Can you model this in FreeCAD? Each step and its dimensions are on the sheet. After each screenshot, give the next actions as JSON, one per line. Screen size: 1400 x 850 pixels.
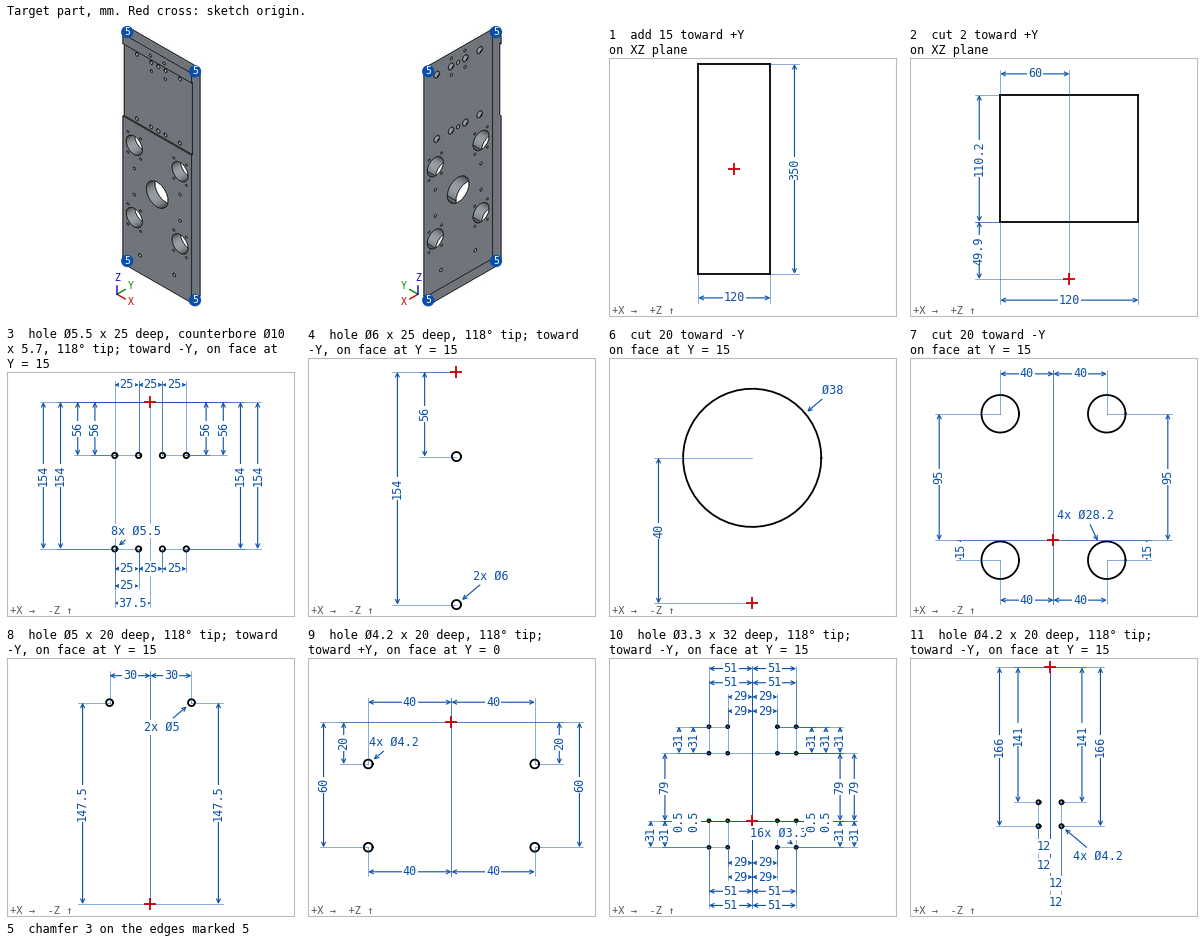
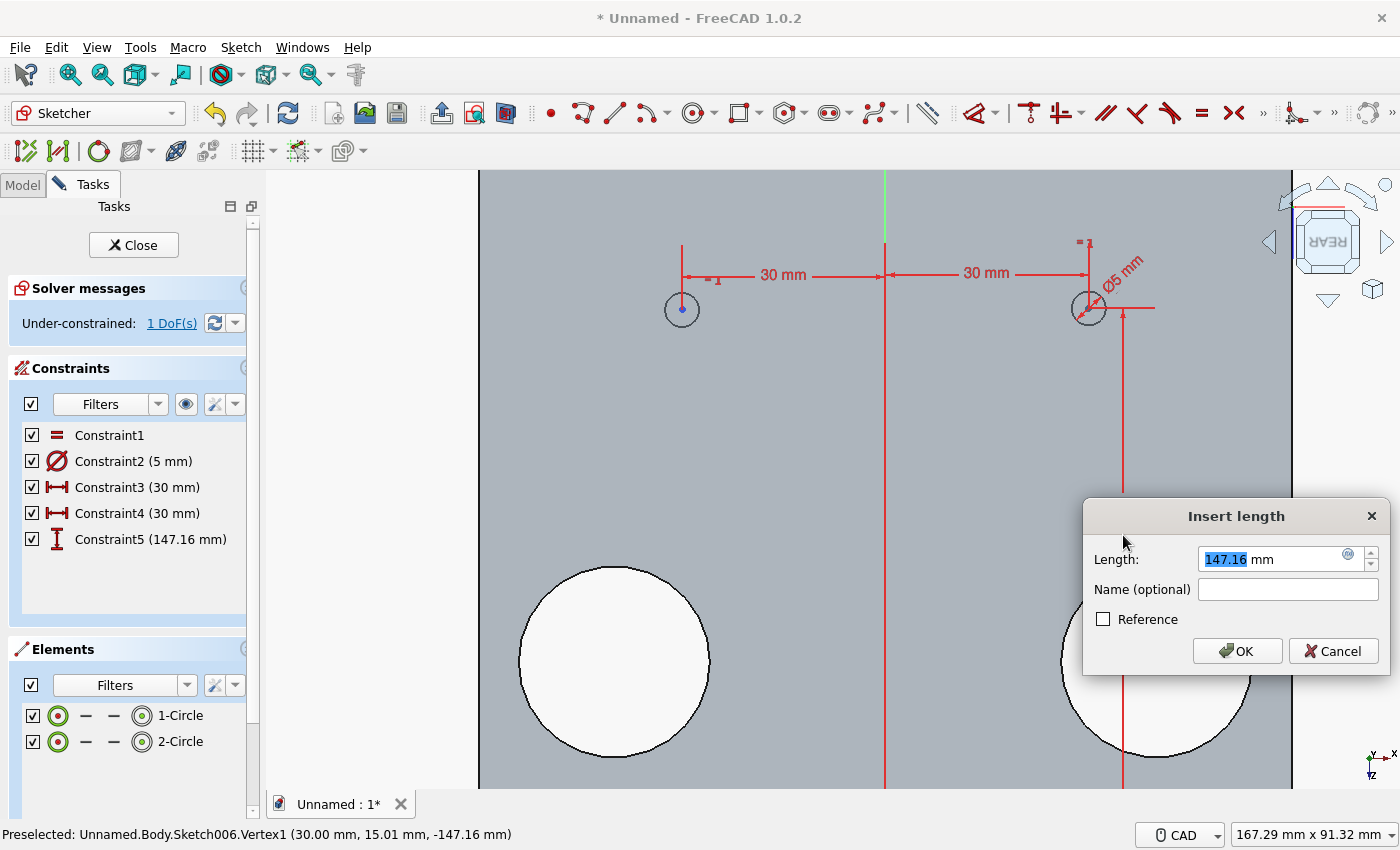
{"action": "type", "text": "147.5"}
{"action": "key", "text": "Return"}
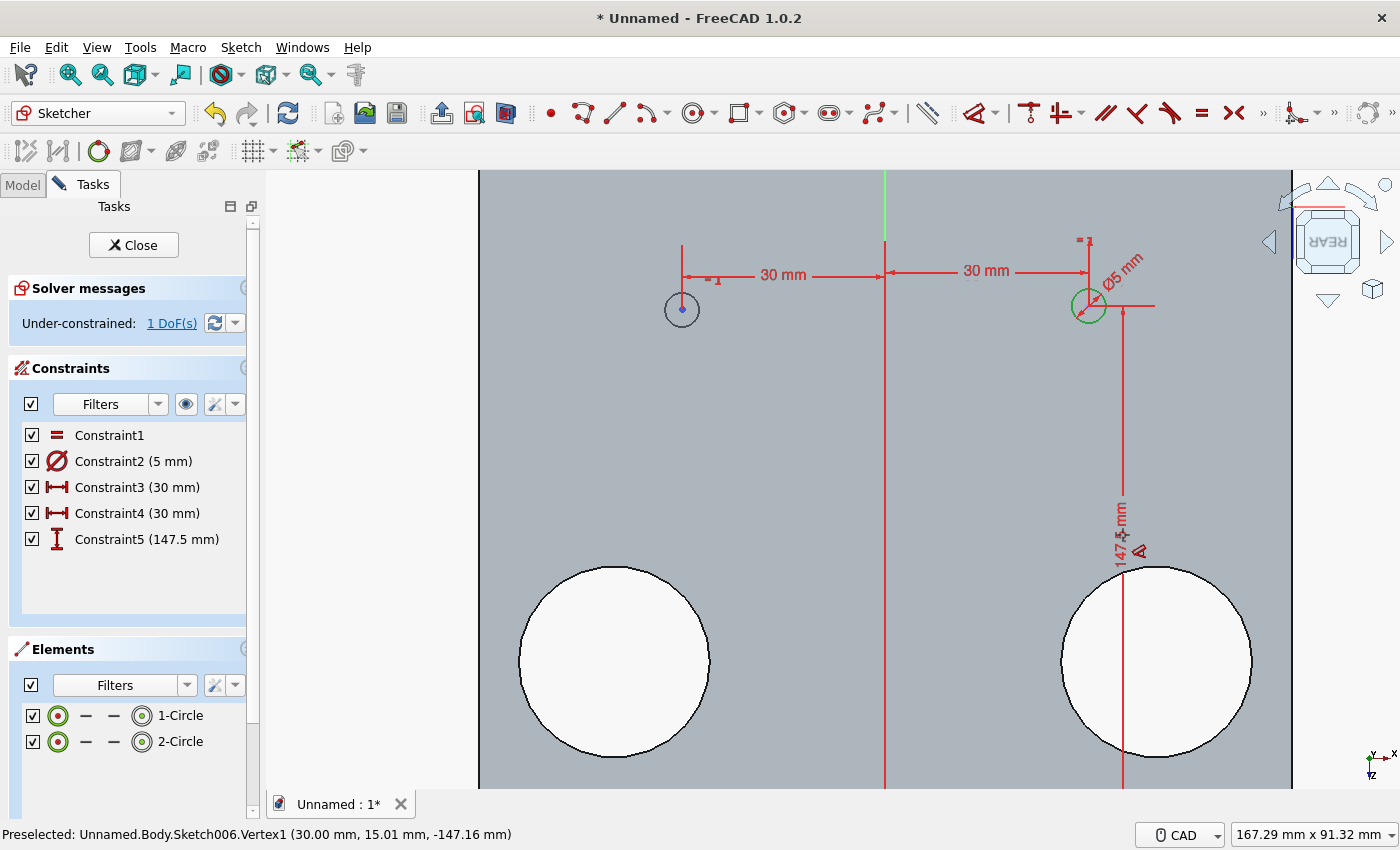
{"action": "left_click", "coordinate": [682, 310]}
{"action": "left_click", "coordinate": [648, 535]}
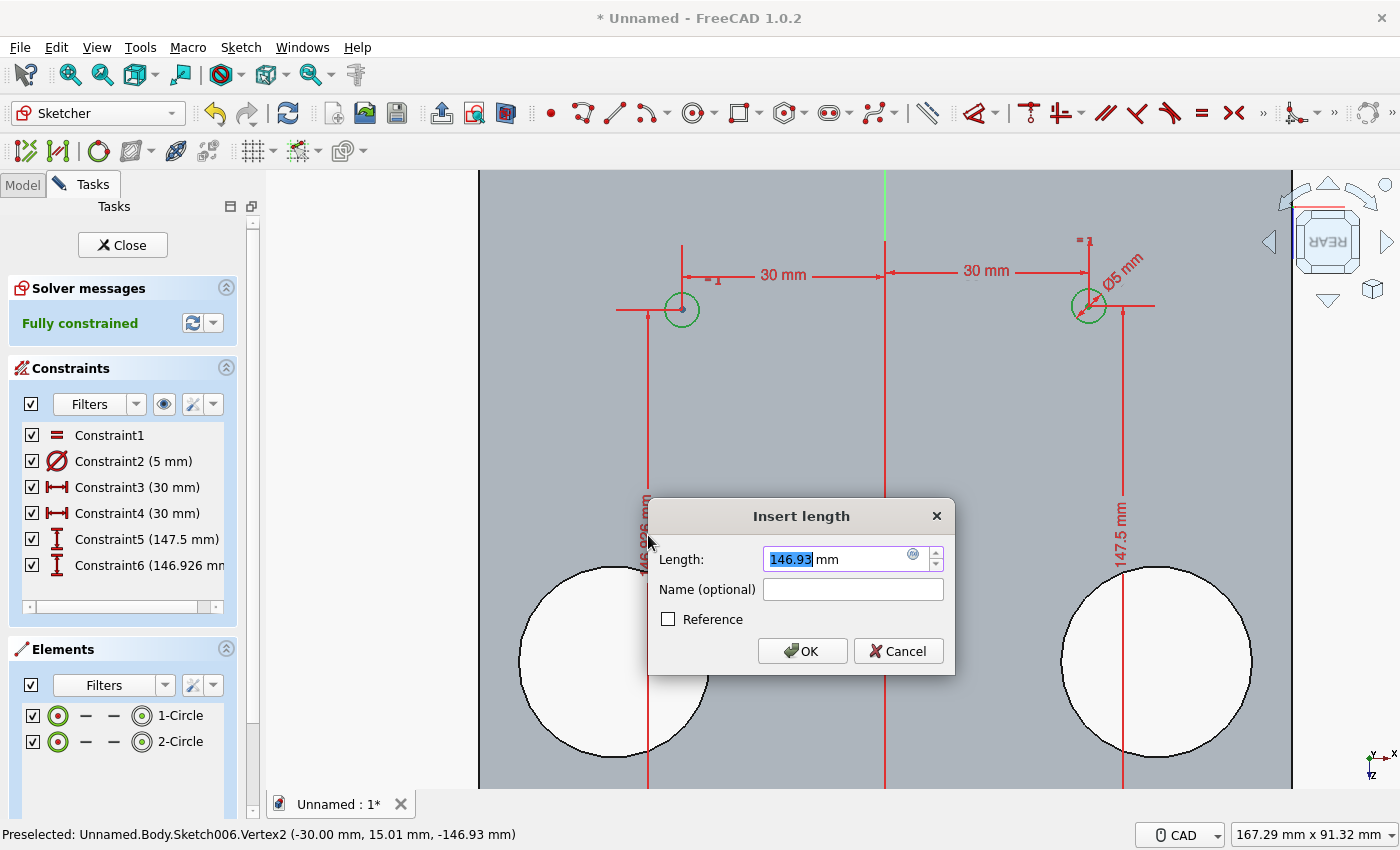
{"action": "type", "text": "147.5"}
{"action": "key", "text": "Return"}
{"action": "key", "text": "Escape"}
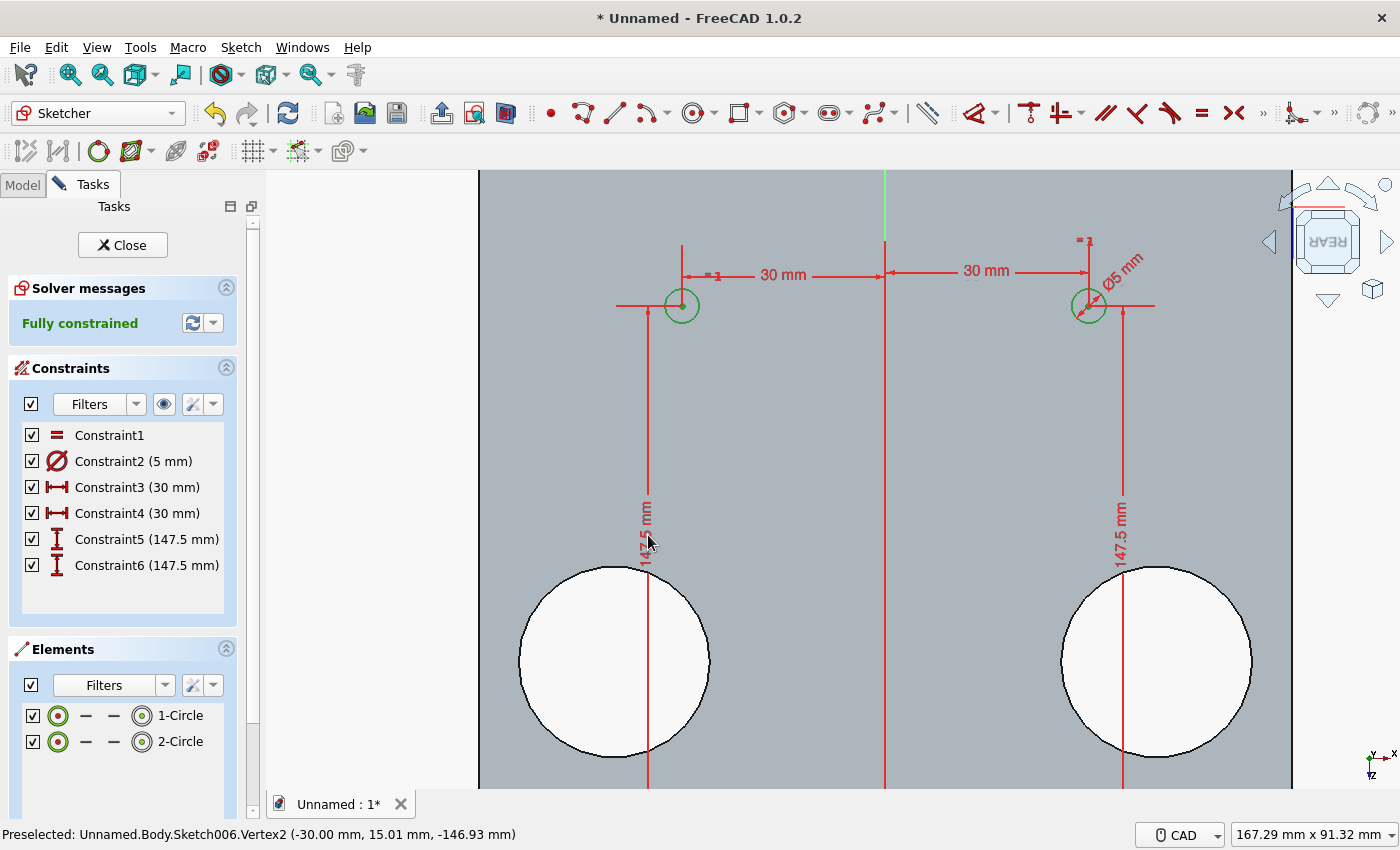
{"action": "left_click", "coordinate": [123, 245]}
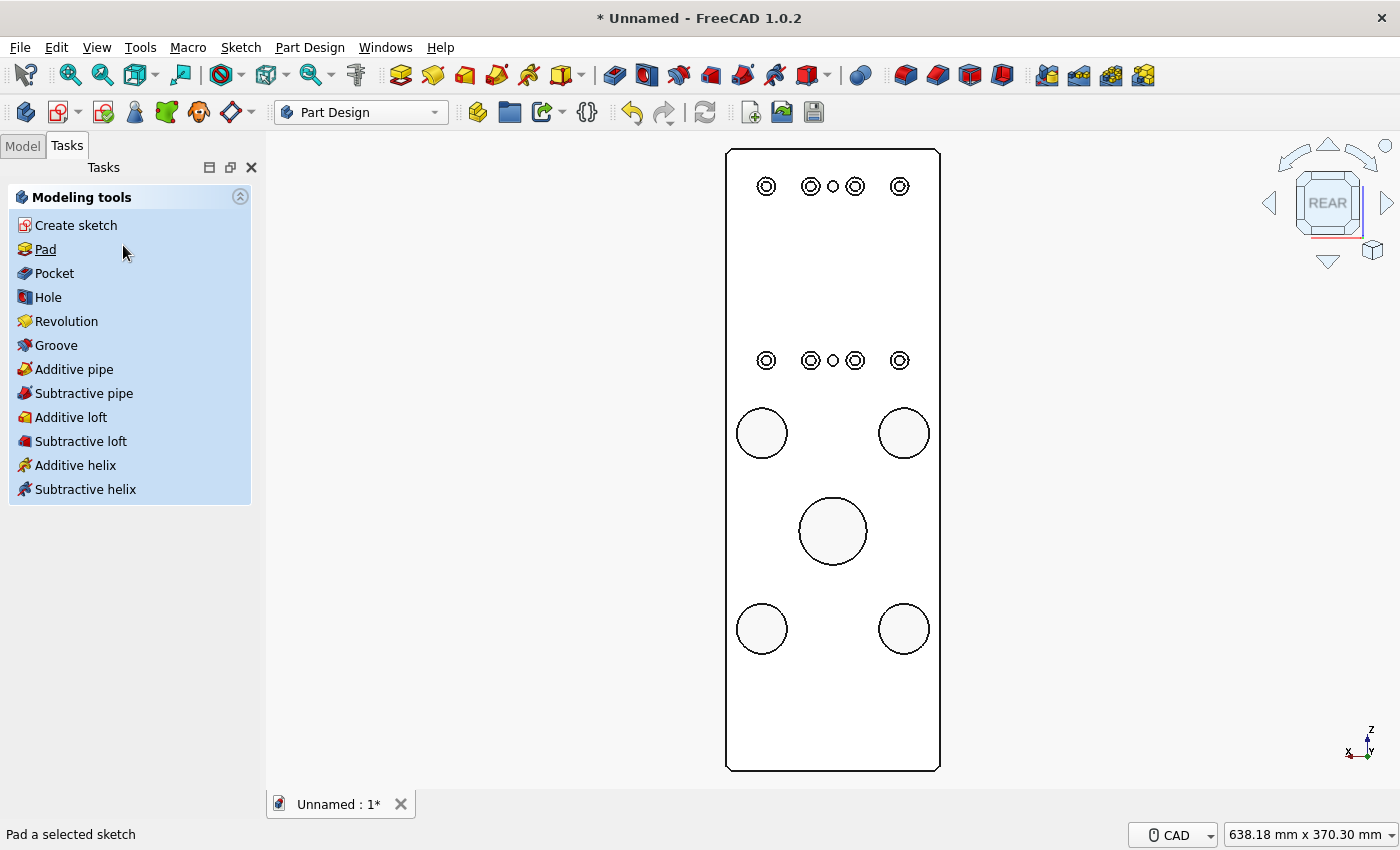
{"action": "left_click", "coordinate": [648, 76]}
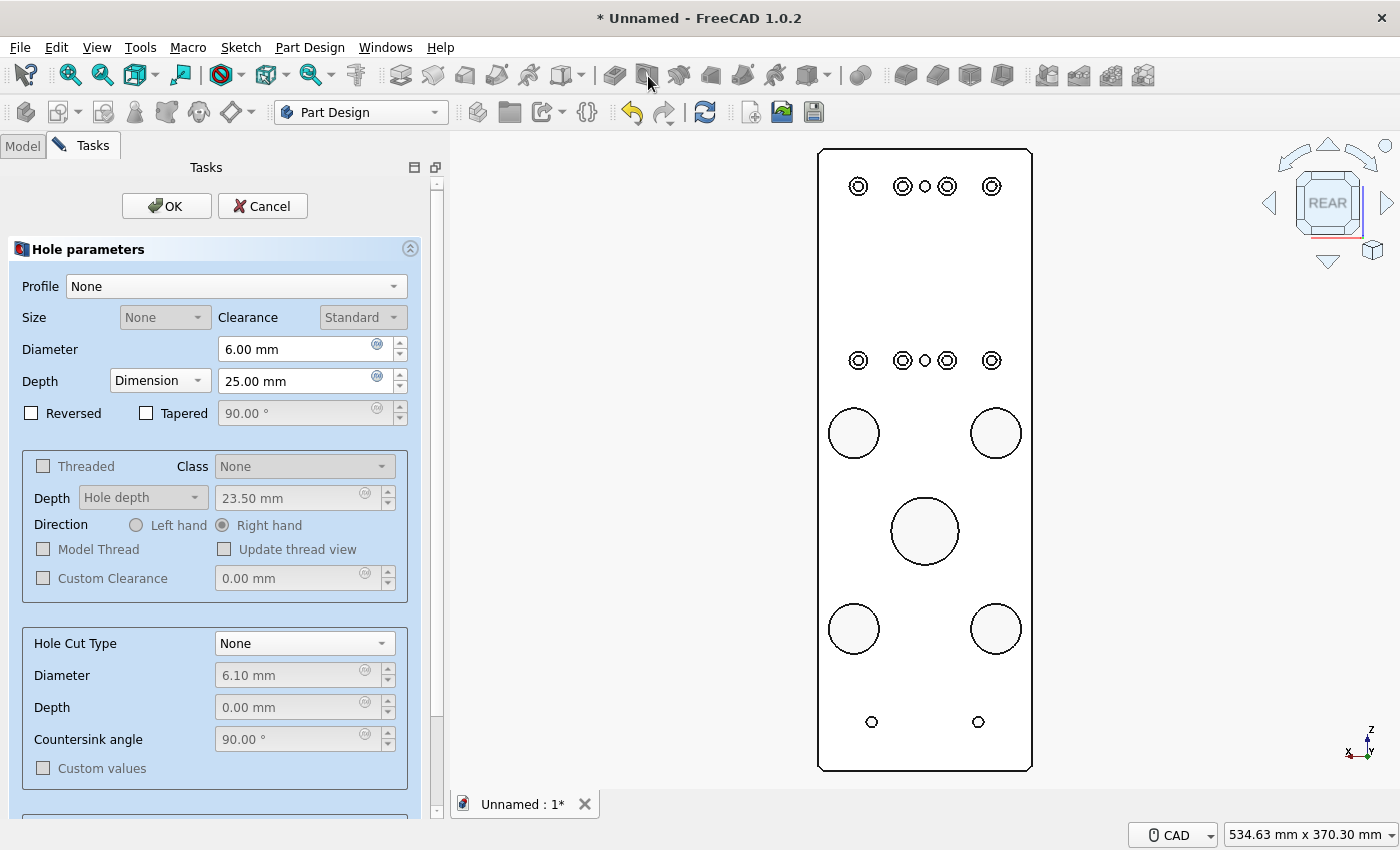
{"action": "triple_click", "coordinate": [305, 349]}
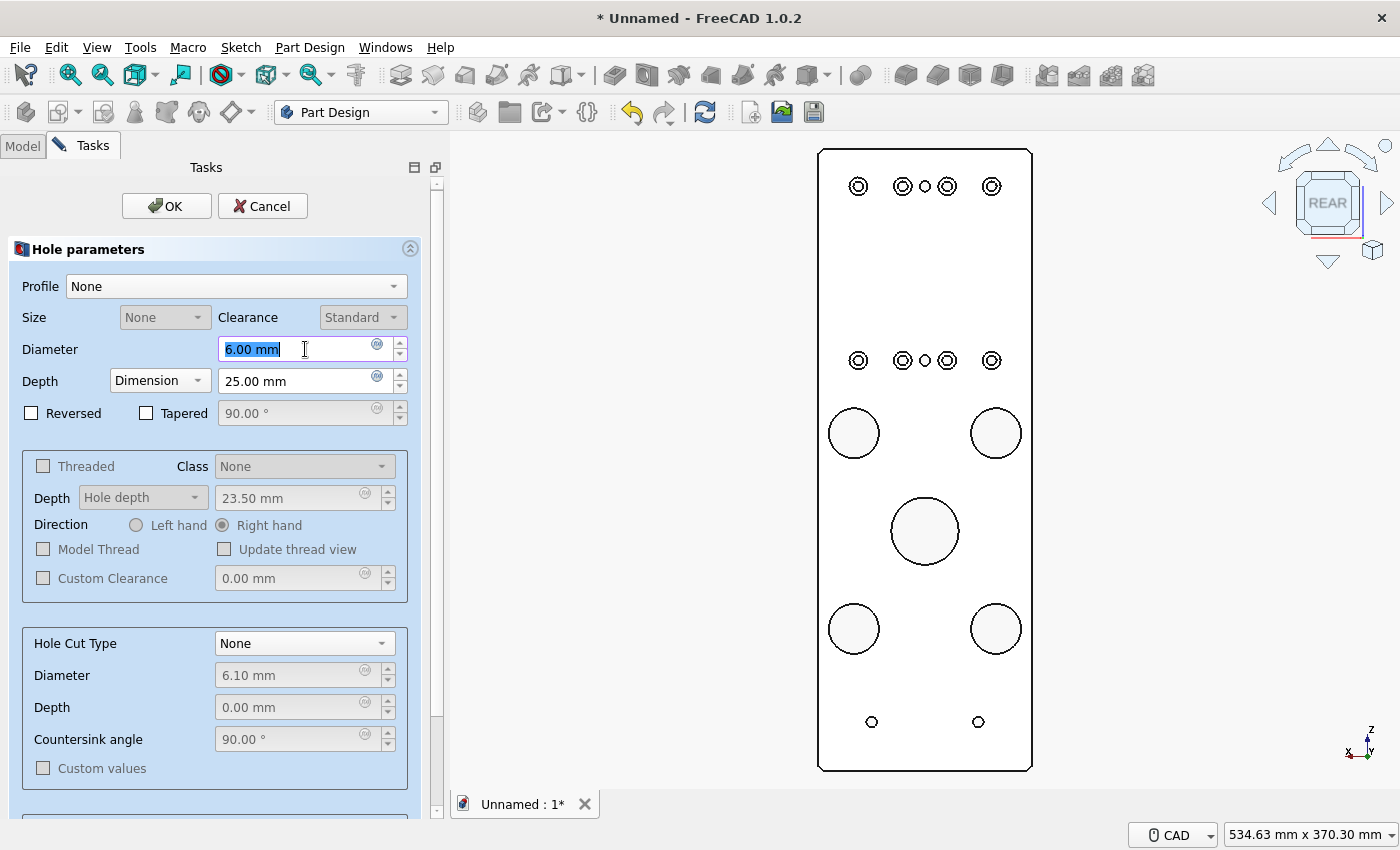
{"action": "type", "text": "5"}
{"action": "key", "text": "Tab"}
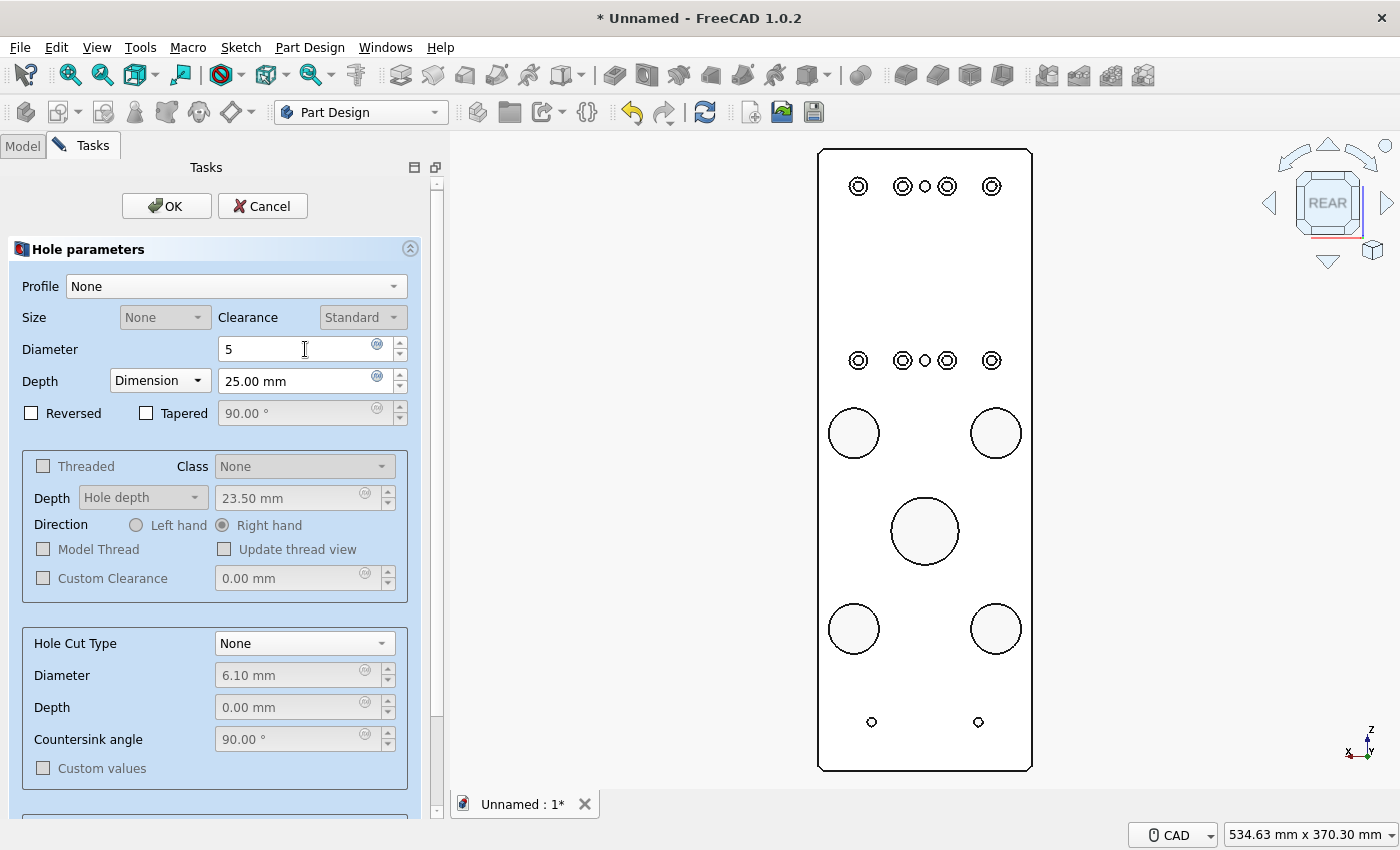
{"action": "triple_click", "coordinate": [305, 381]}